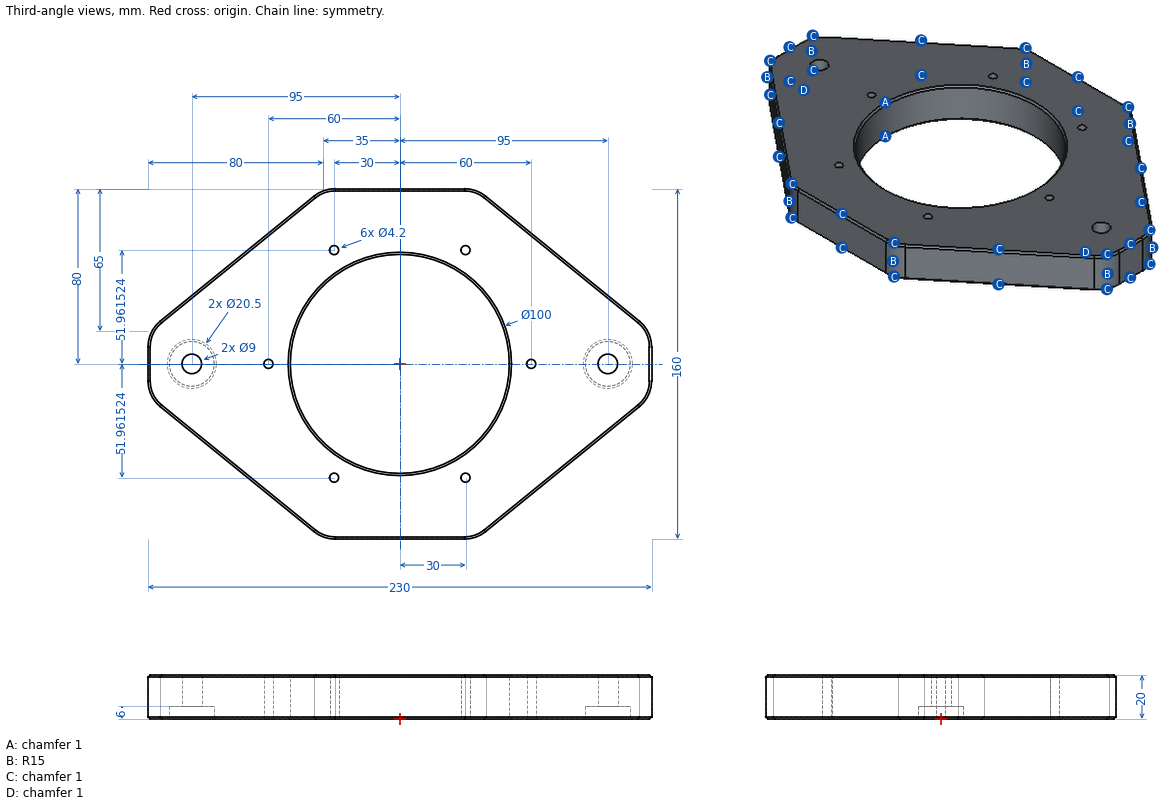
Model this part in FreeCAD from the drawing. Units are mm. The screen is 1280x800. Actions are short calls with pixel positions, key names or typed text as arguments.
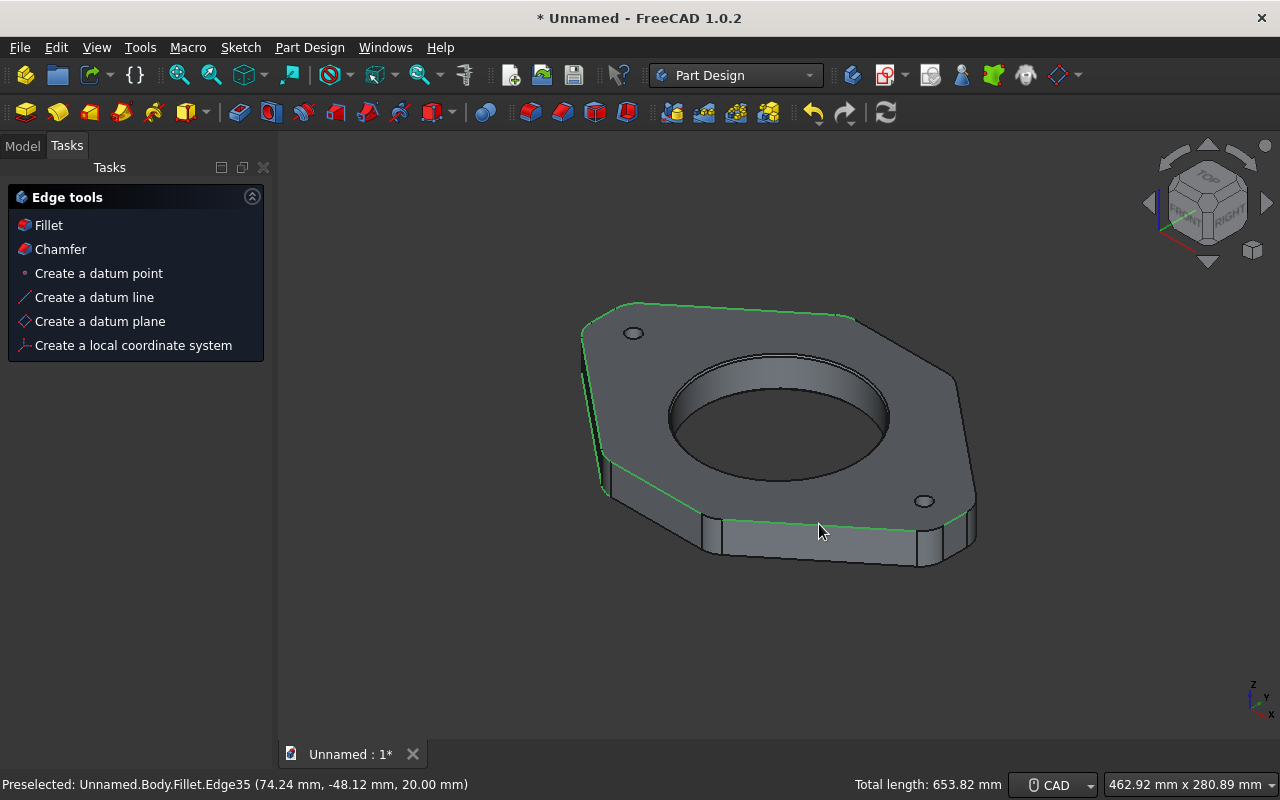
click(711, 517, ctrl)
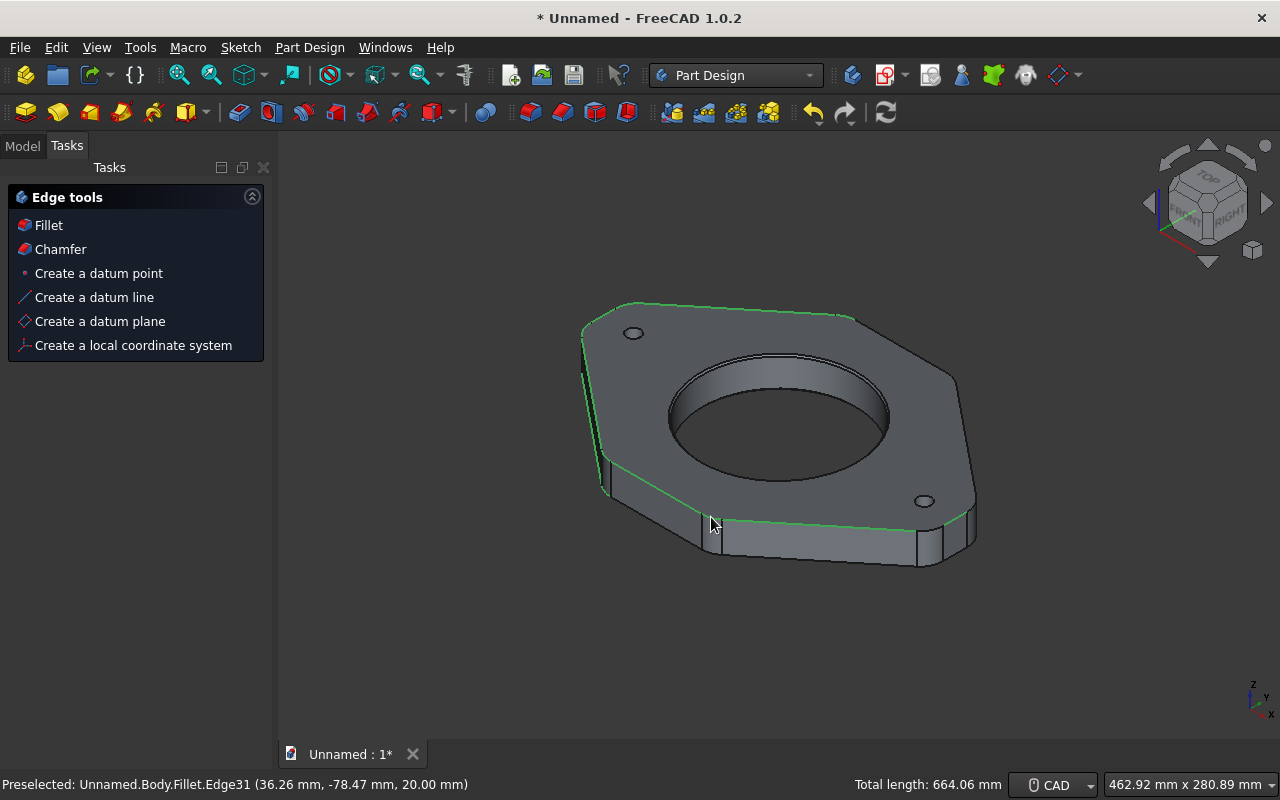
click(931, 529, ctrl)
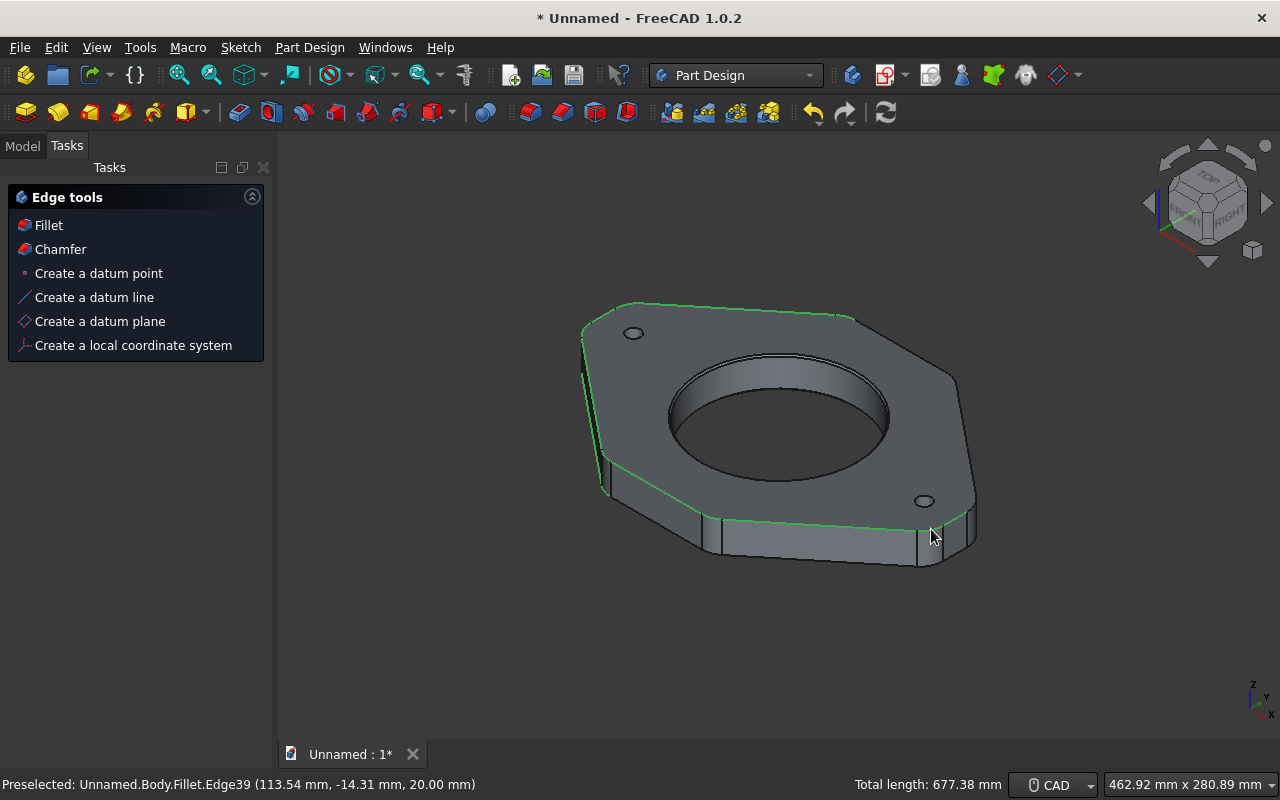
click(975, 504, ctrl)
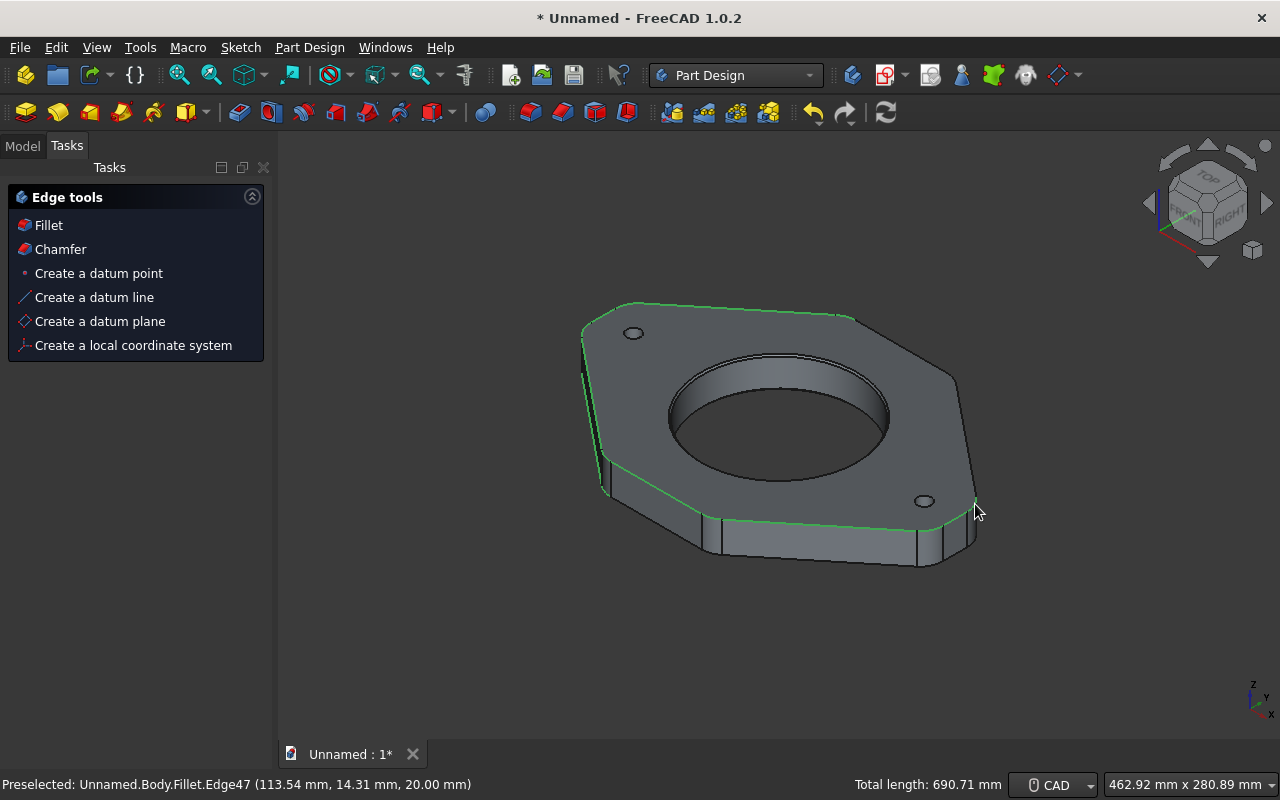
click(950, 374, ctrl)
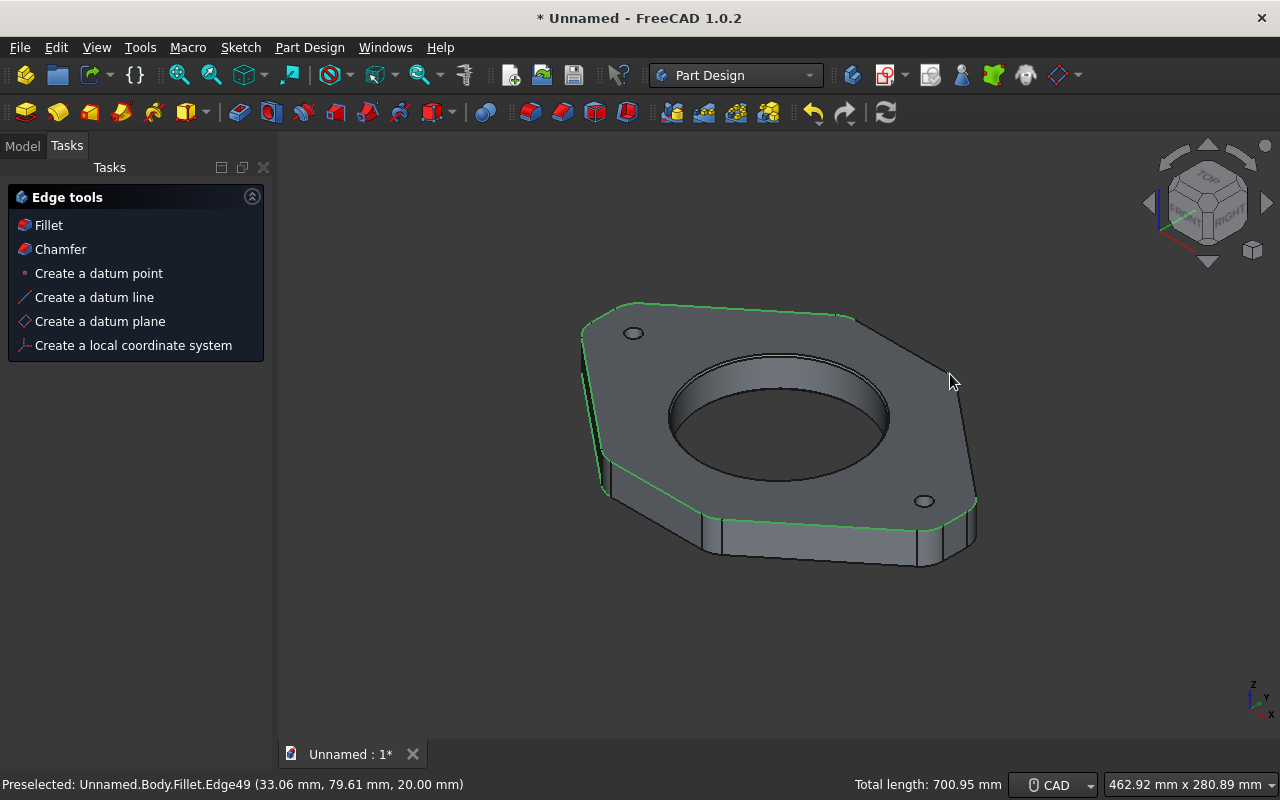
click(705, 550, ctrl)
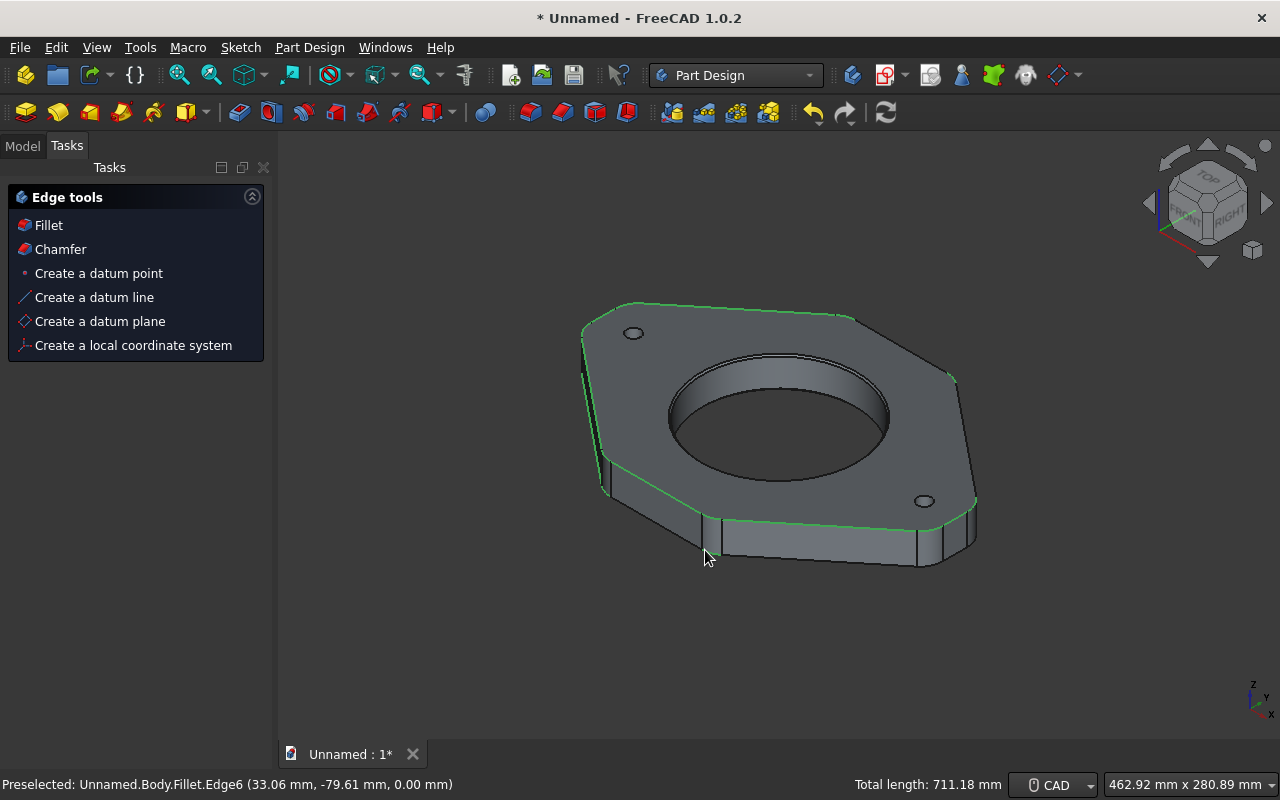
click(934, 564, ctrl)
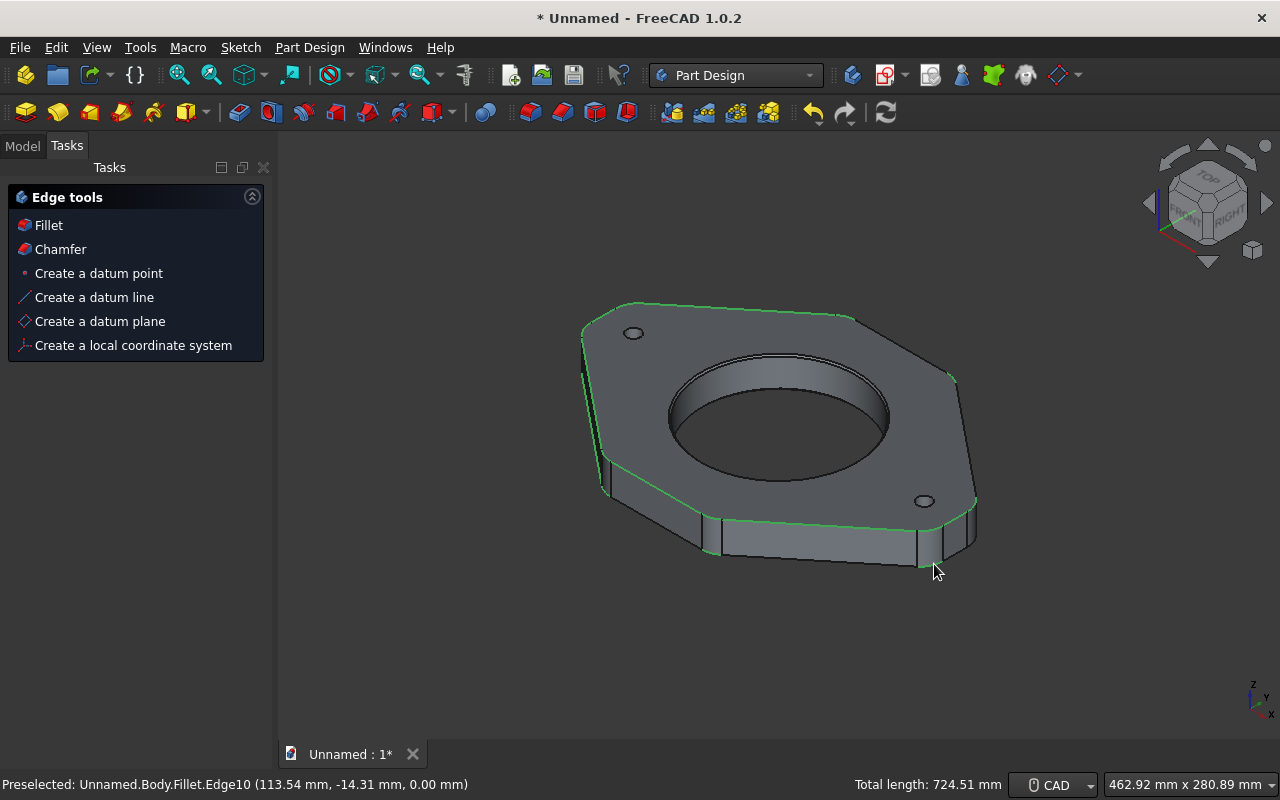
click(974, 541, ctrl)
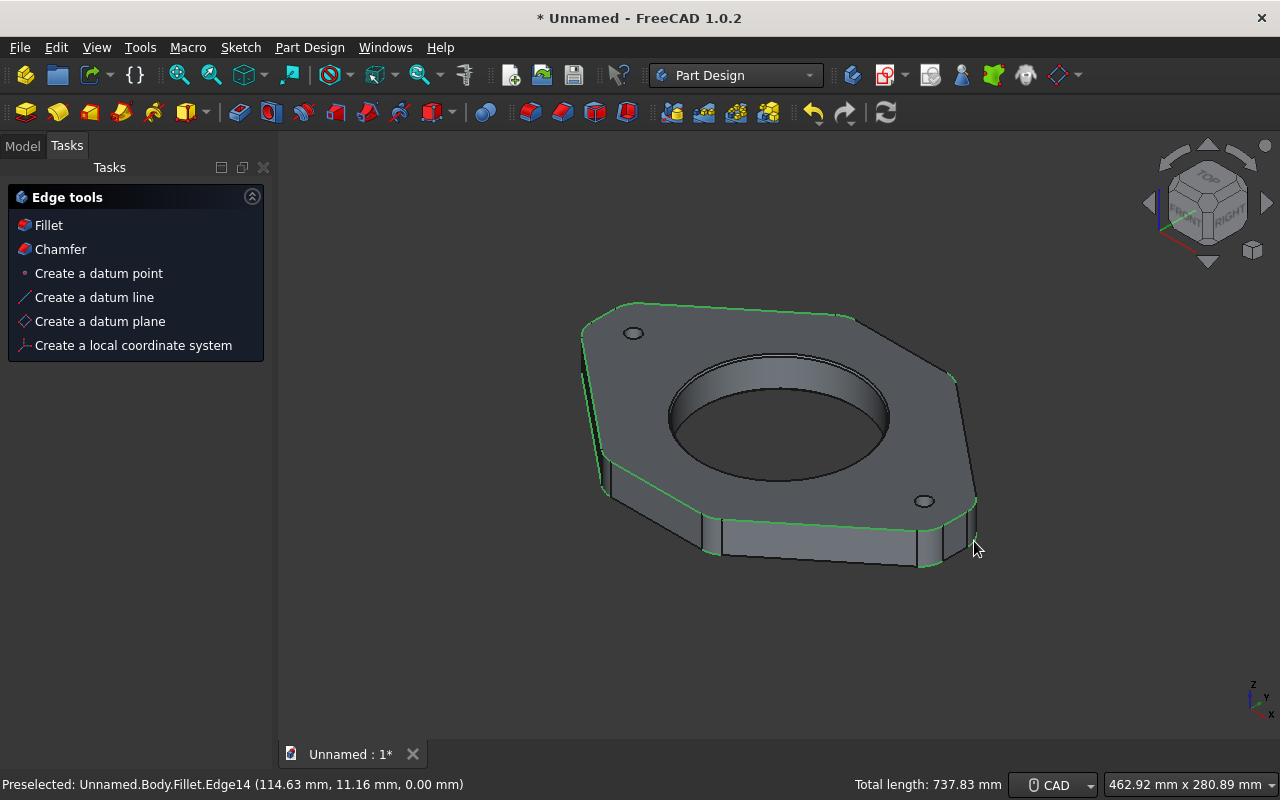
key(2)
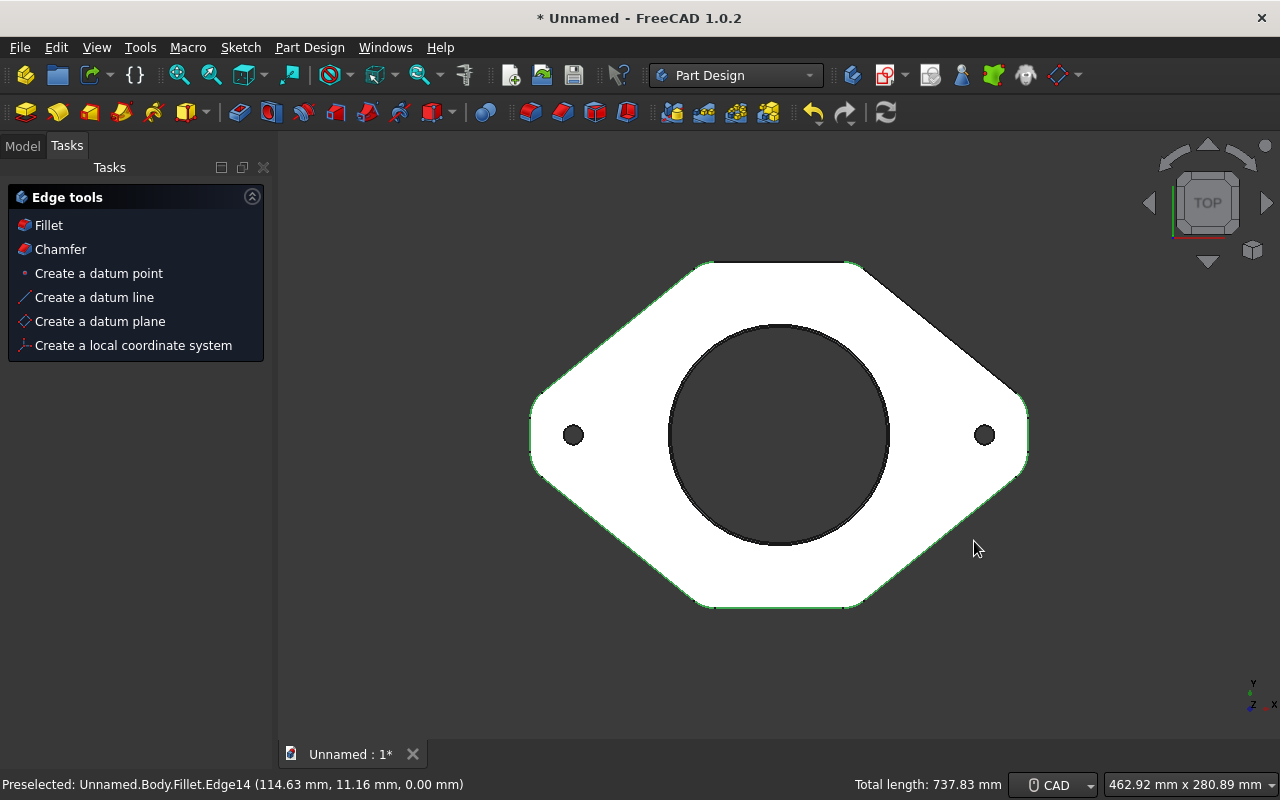
click(940, 330, ctrl)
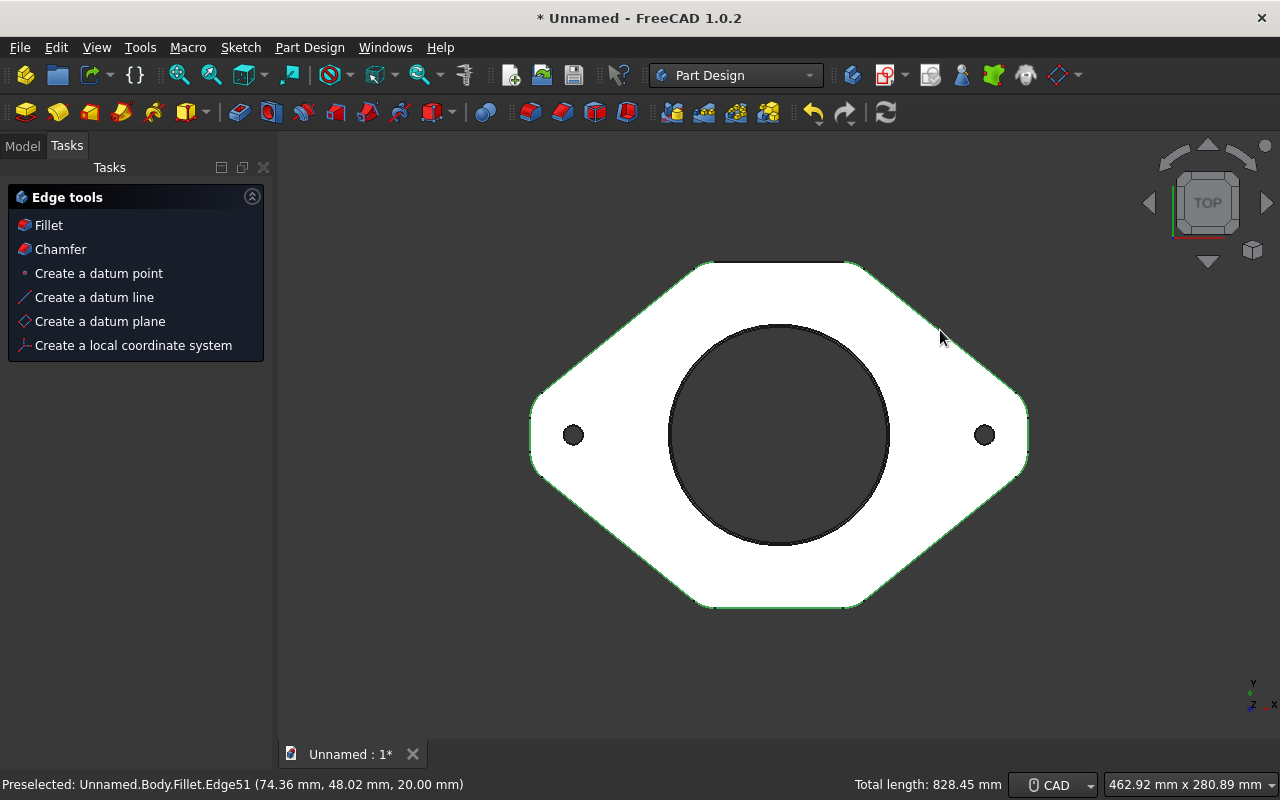
click(779, 261, ctrl)